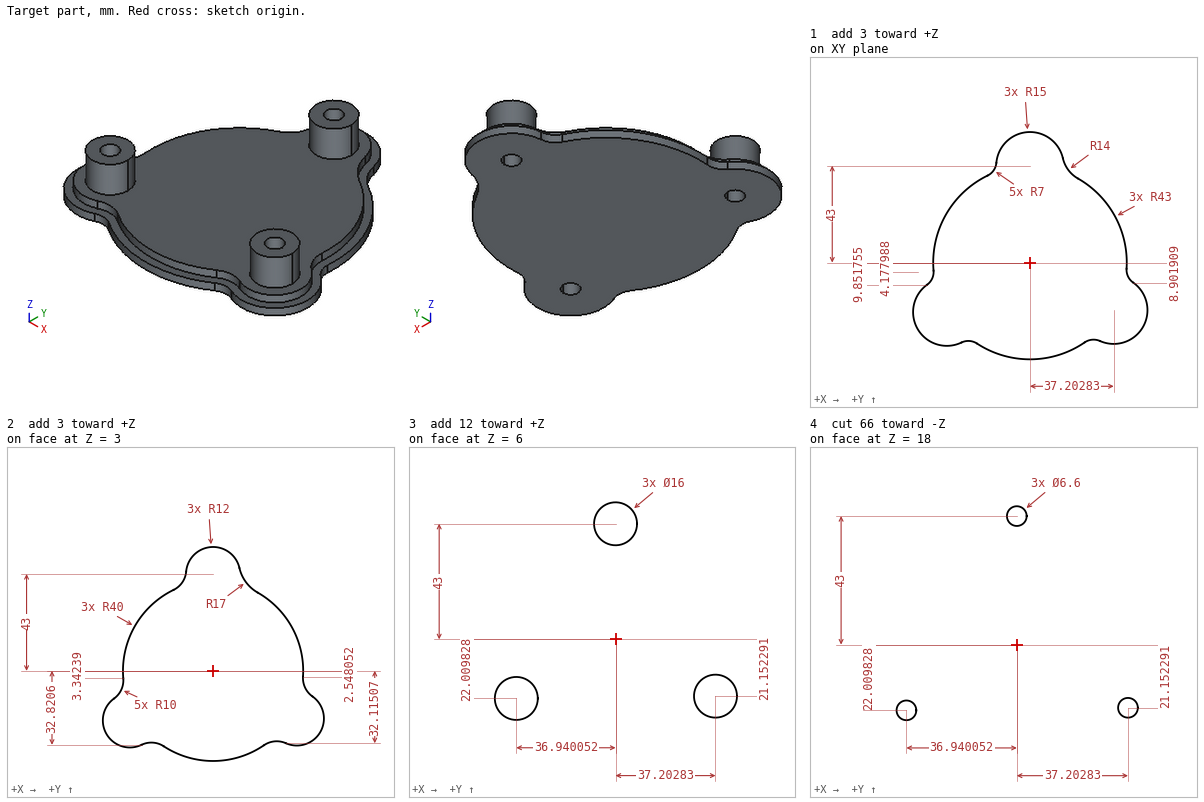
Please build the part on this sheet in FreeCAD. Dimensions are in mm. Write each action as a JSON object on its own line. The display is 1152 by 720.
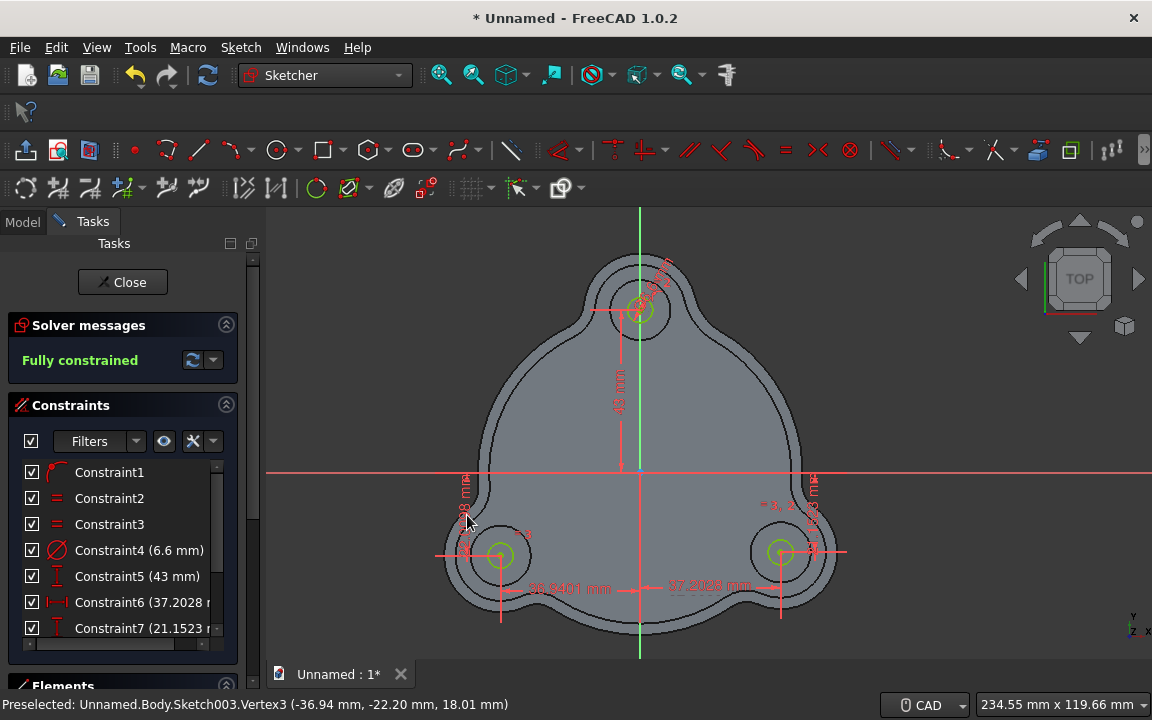
{"action": "left_click", "coordinate": [123, 282]}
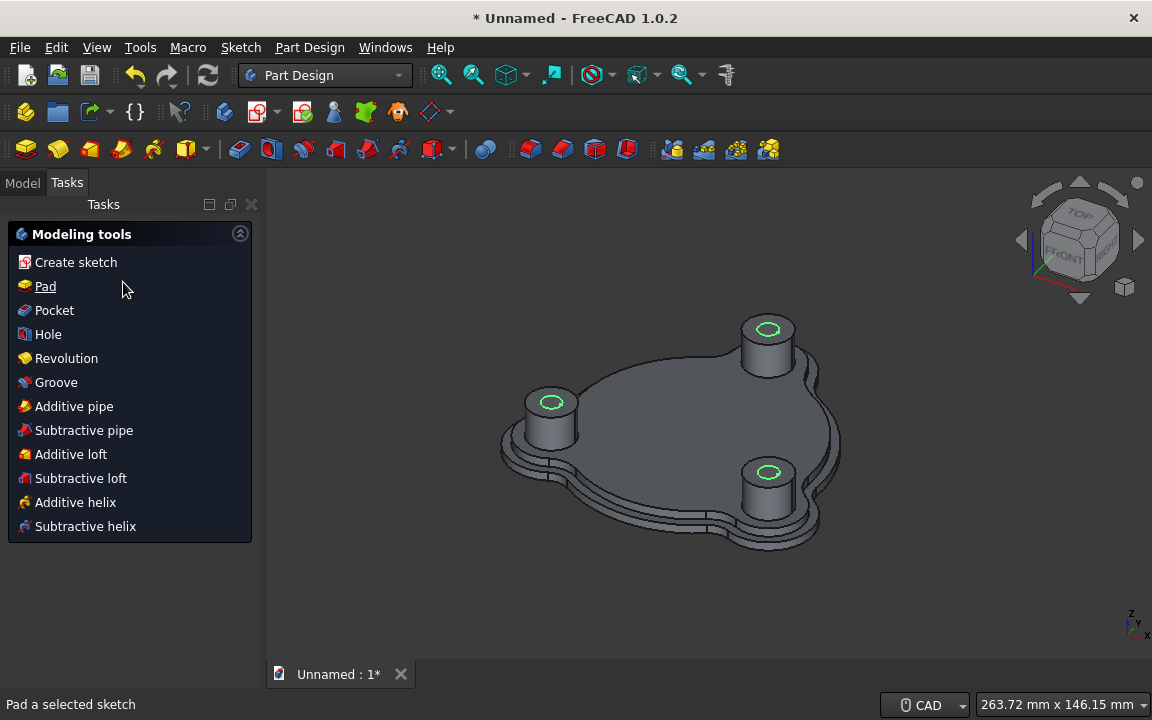
{"action": "left_click", "coordinate": [240, 150]}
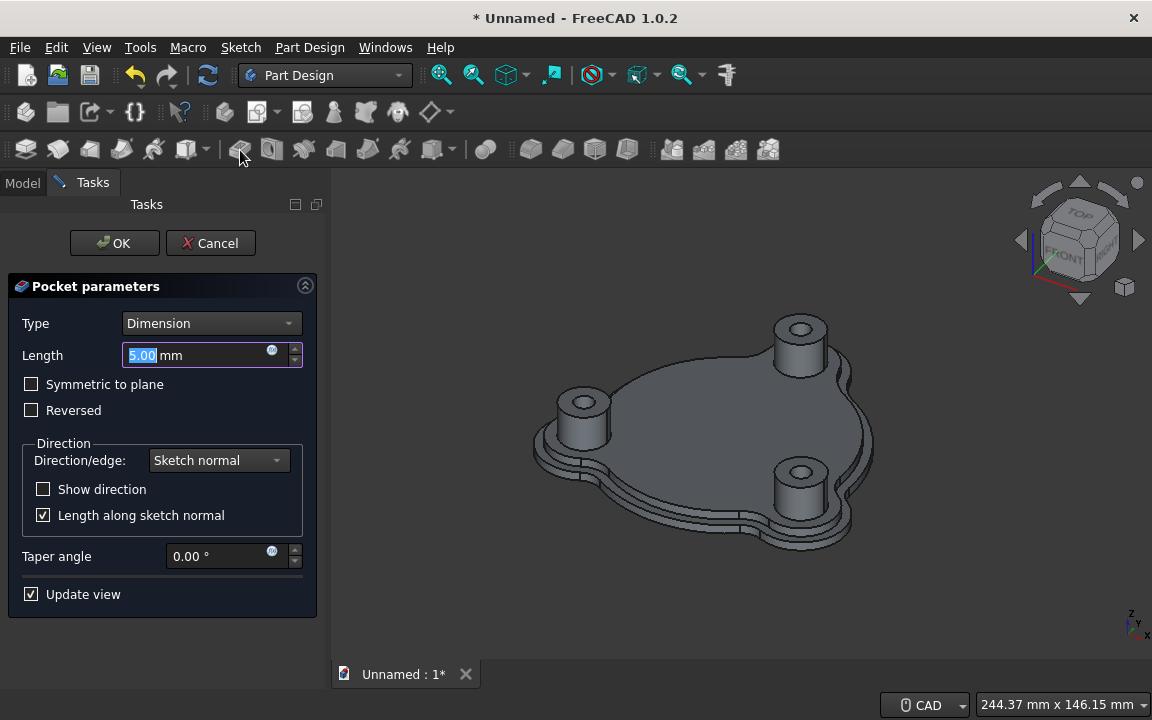
{"action": "type", "text": "66"}
{"action": "key", "text": "Tab"}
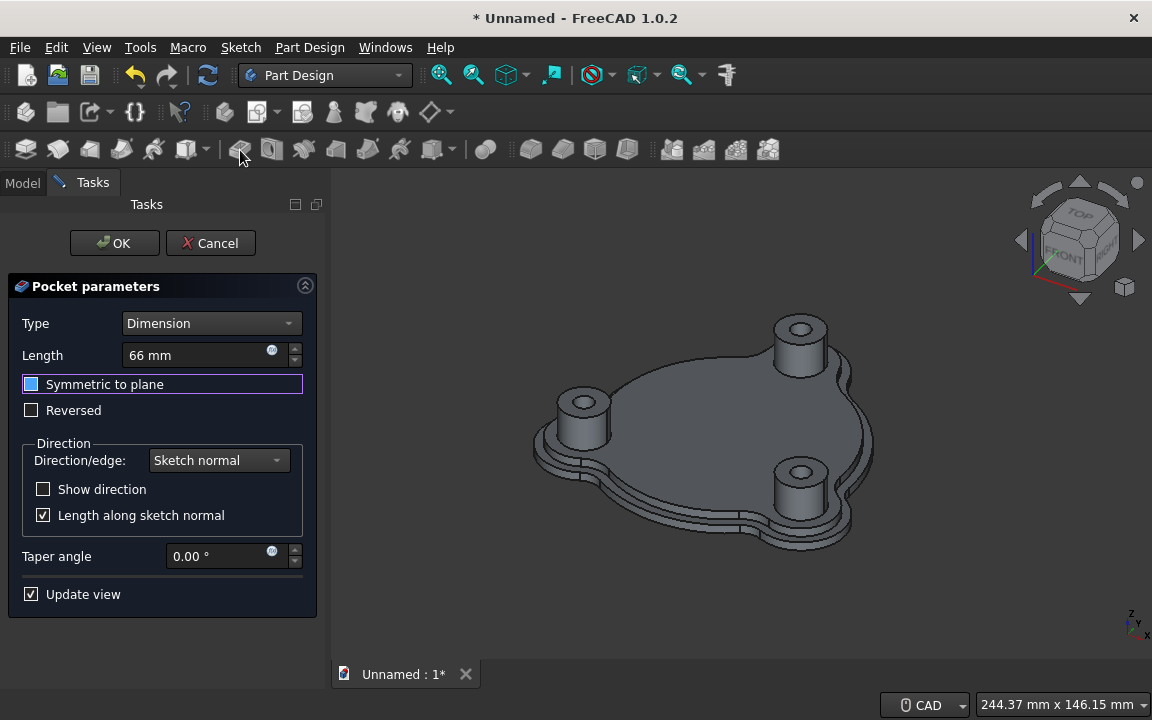
{"action": "left_click", "coordinate": [115, 243]}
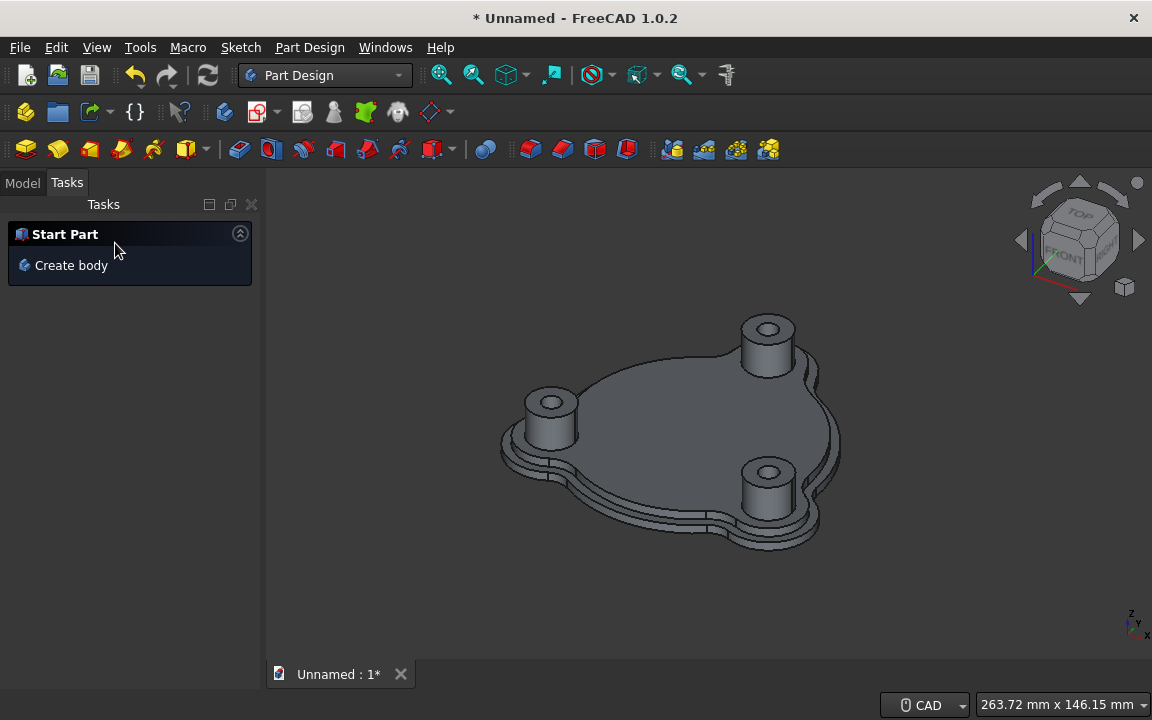
{"action": "key", "text": "0"}